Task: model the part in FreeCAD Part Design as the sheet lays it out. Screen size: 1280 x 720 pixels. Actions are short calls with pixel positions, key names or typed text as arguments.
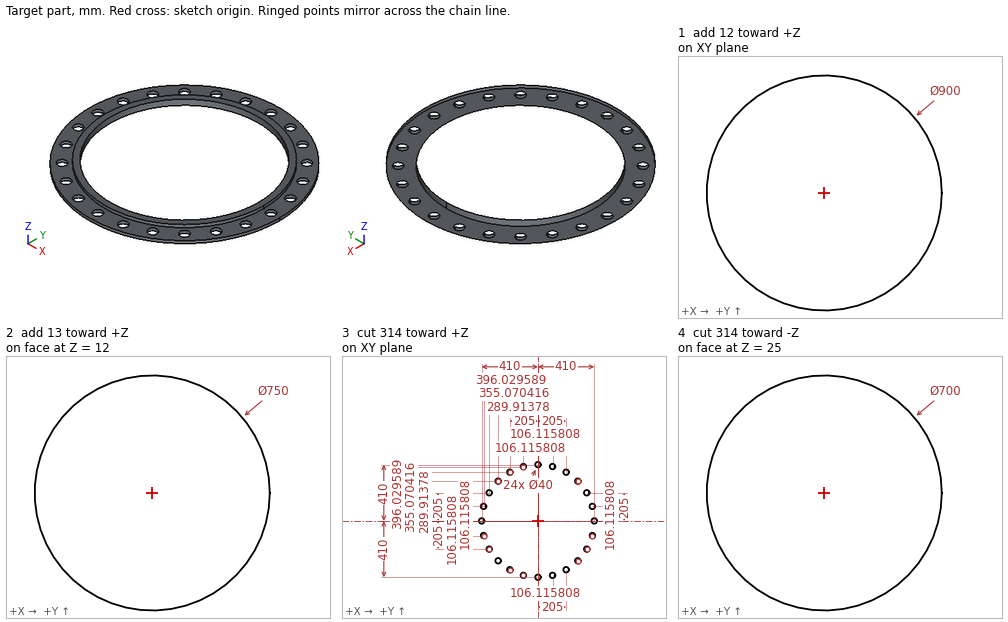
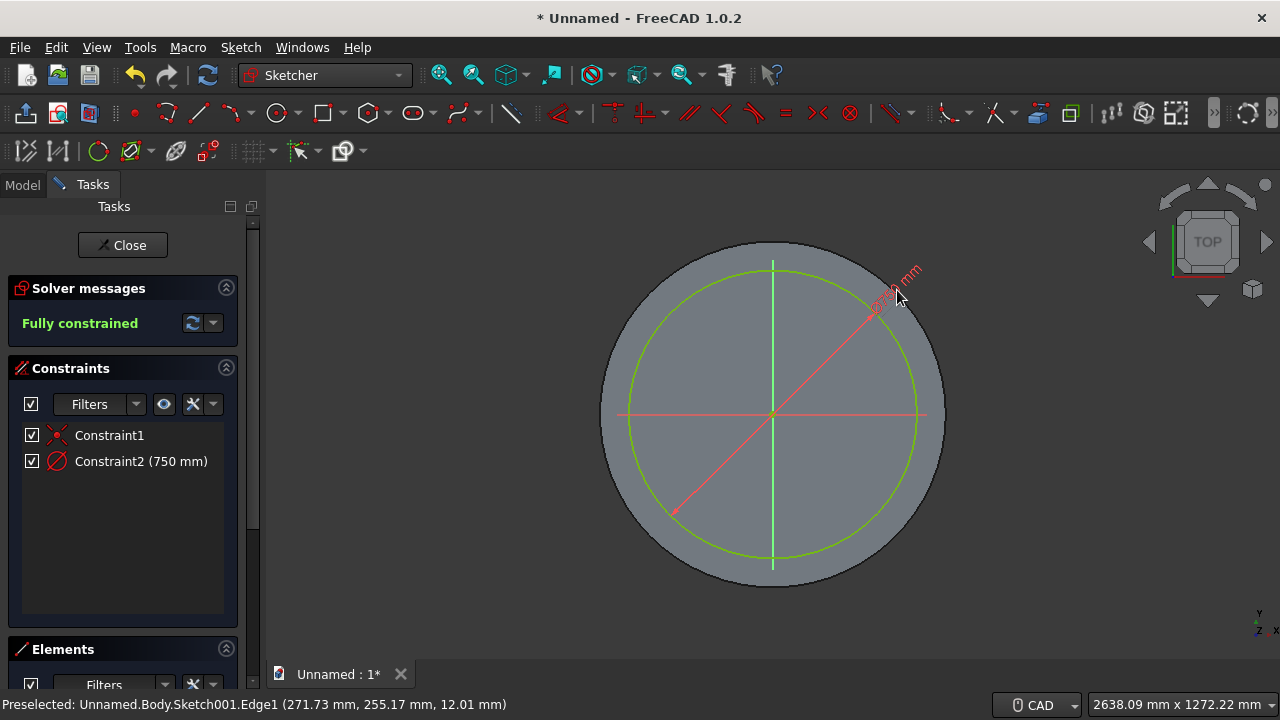
click(123, 245)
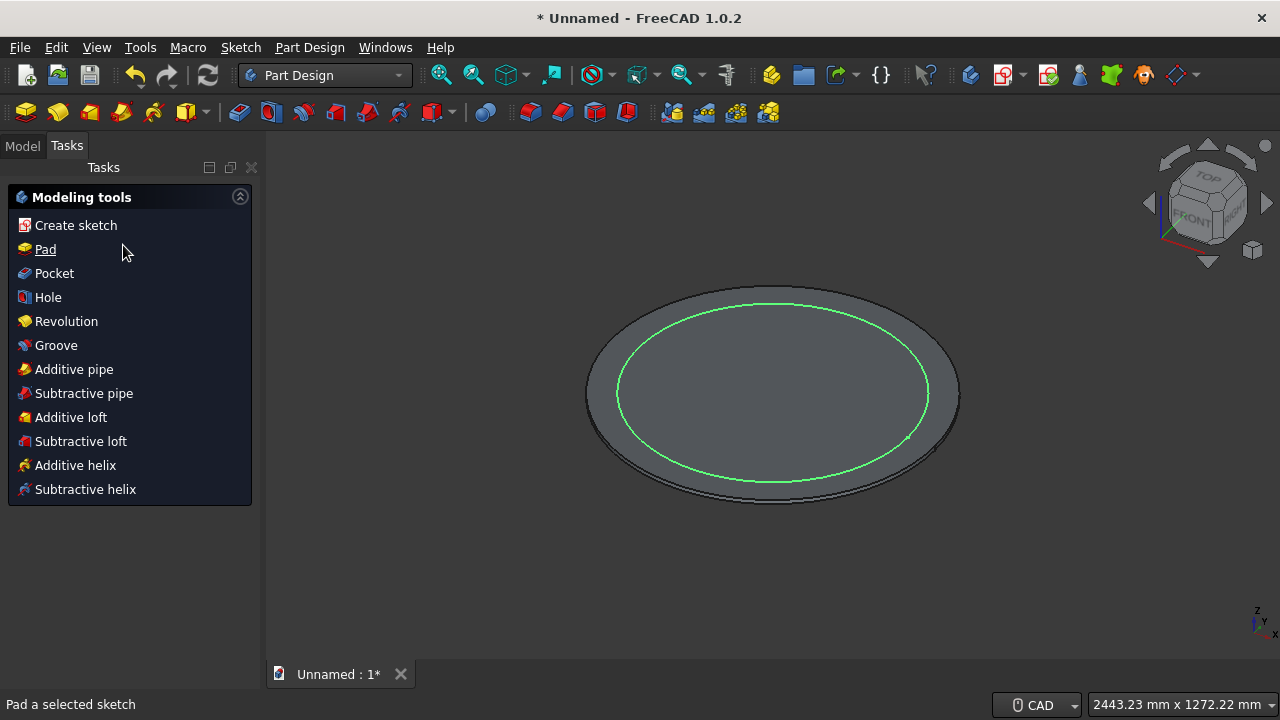
click(26, 112)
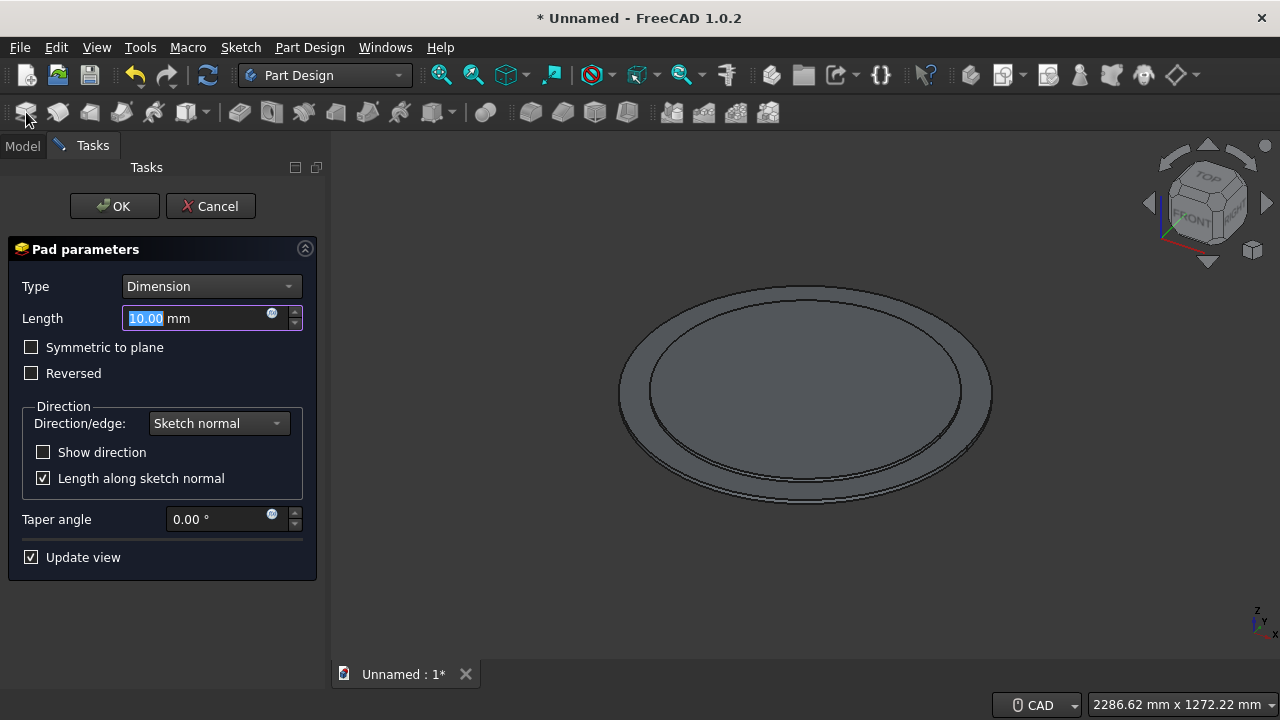
text(13)
key(Tab)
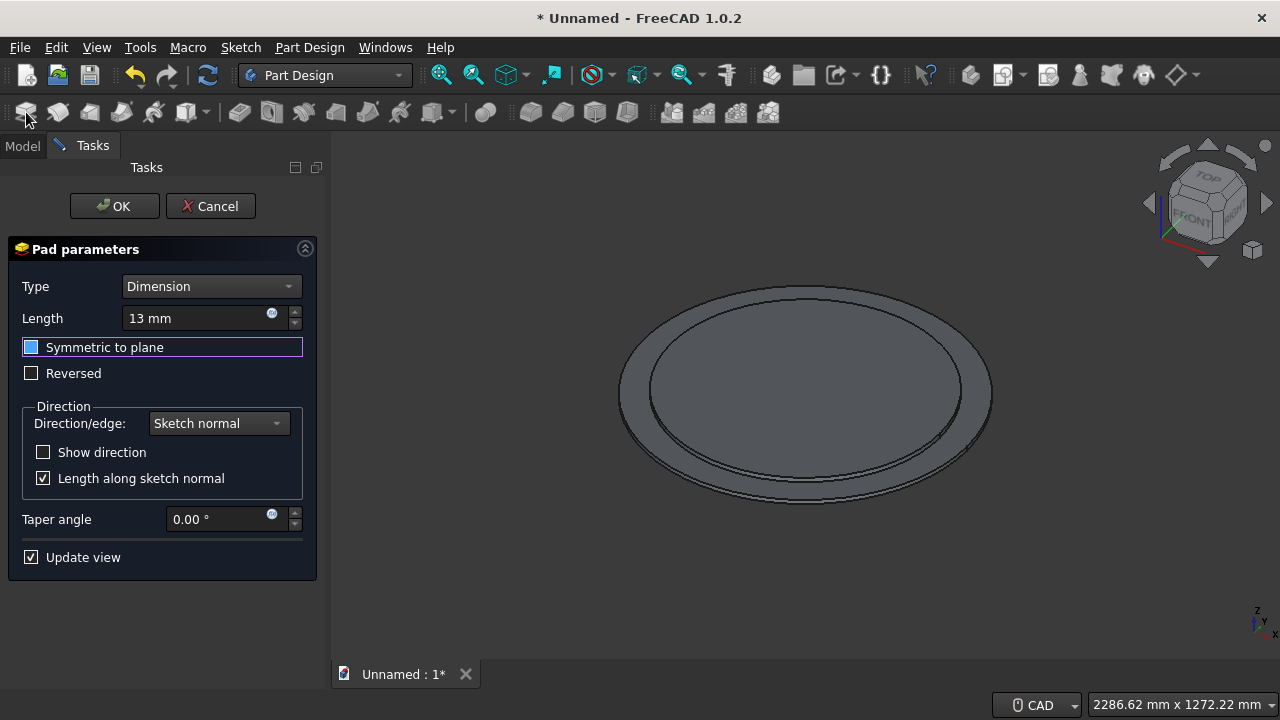
click(115, 206)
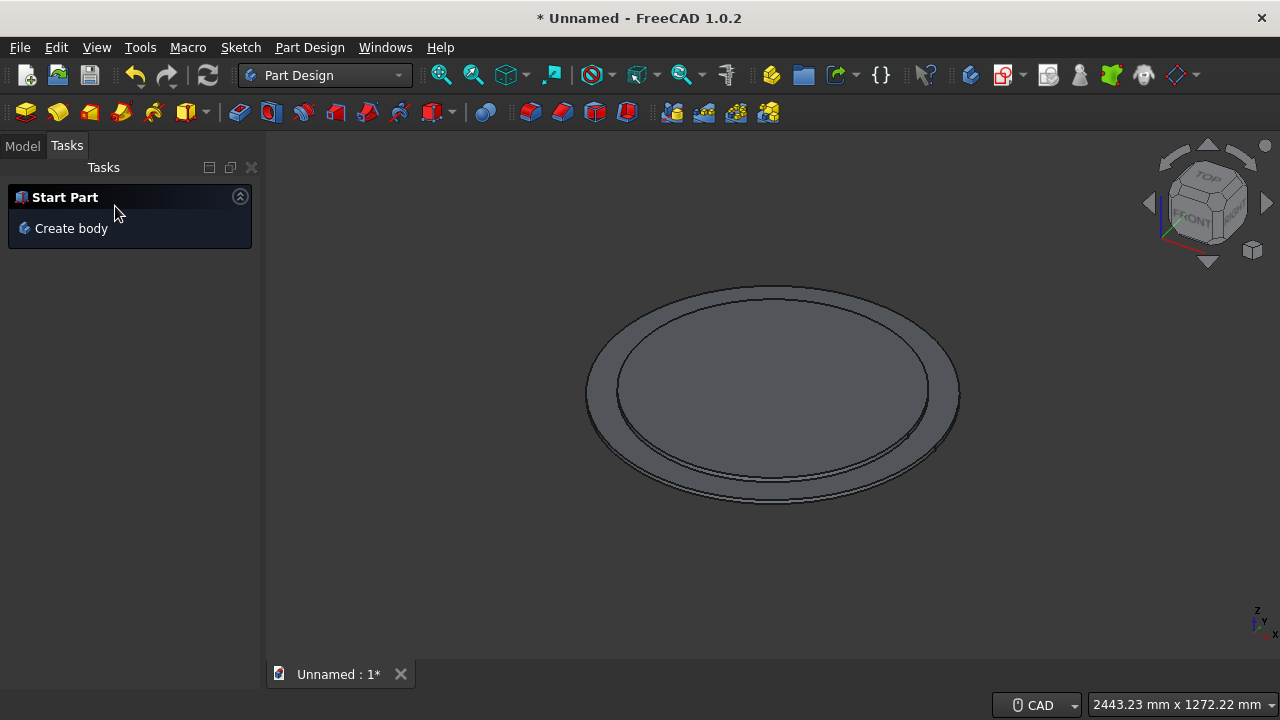
click(1004, 76)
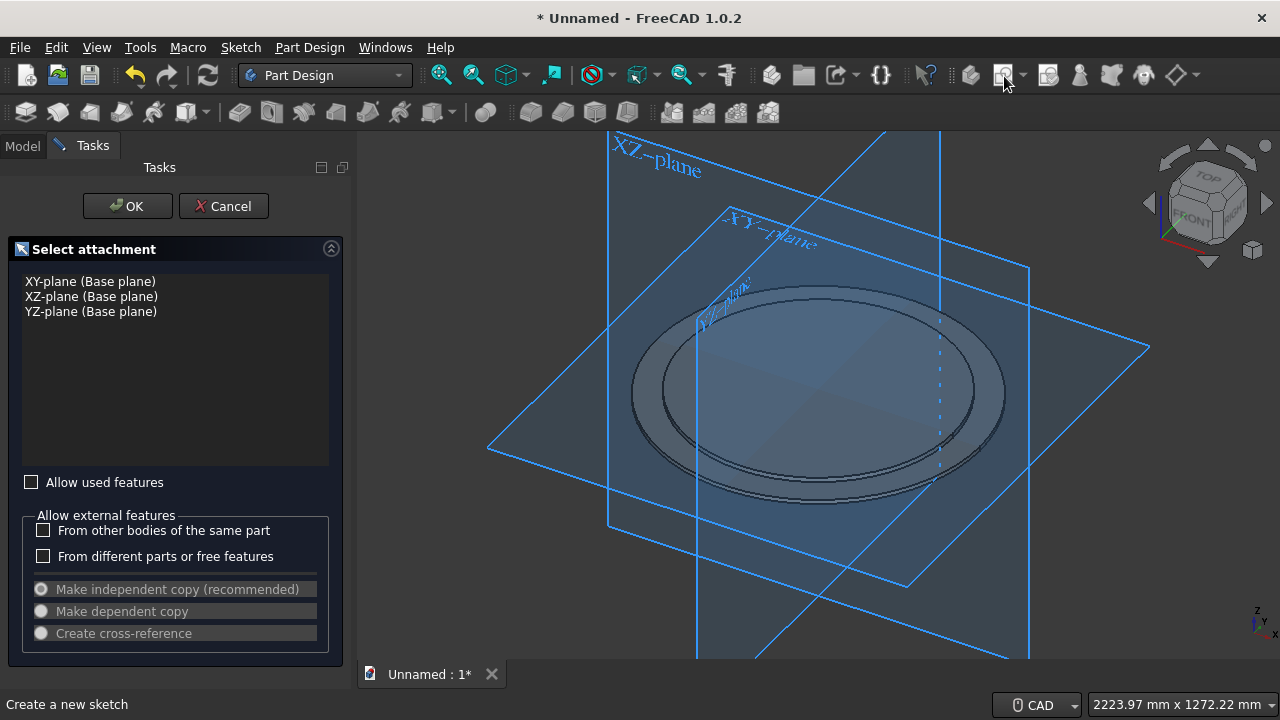
click(82, 282)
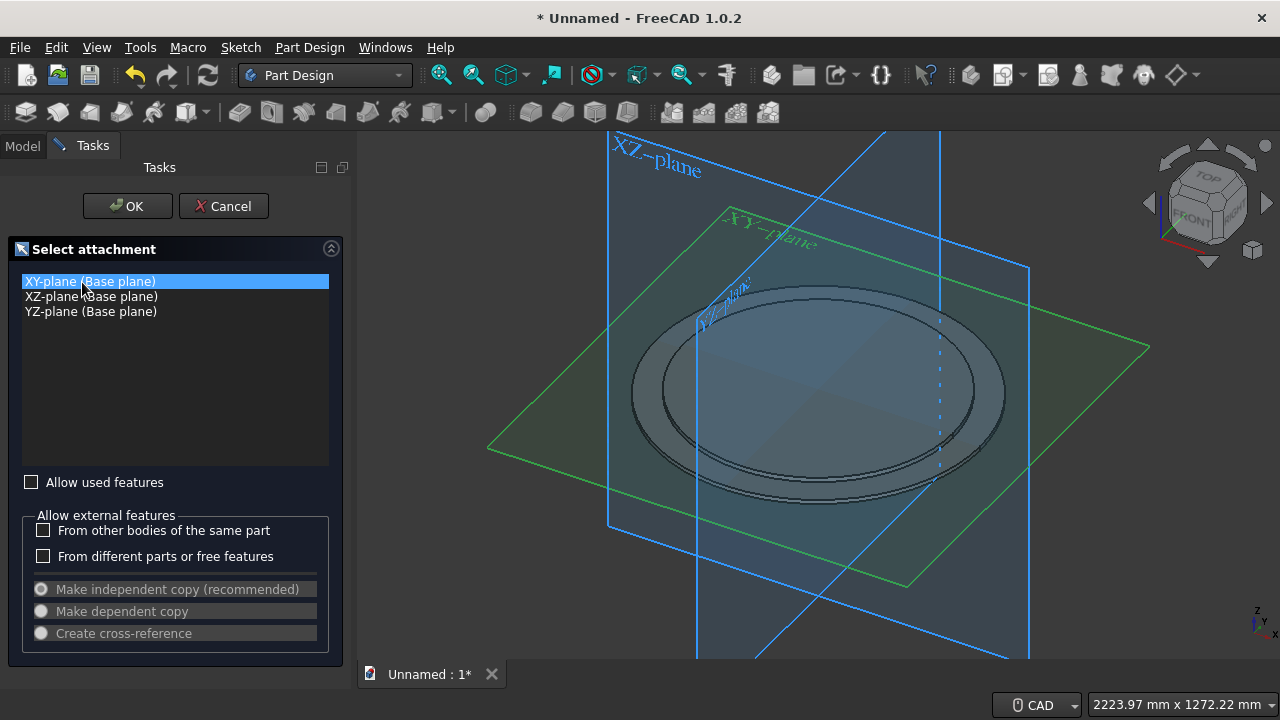
click(128, 206)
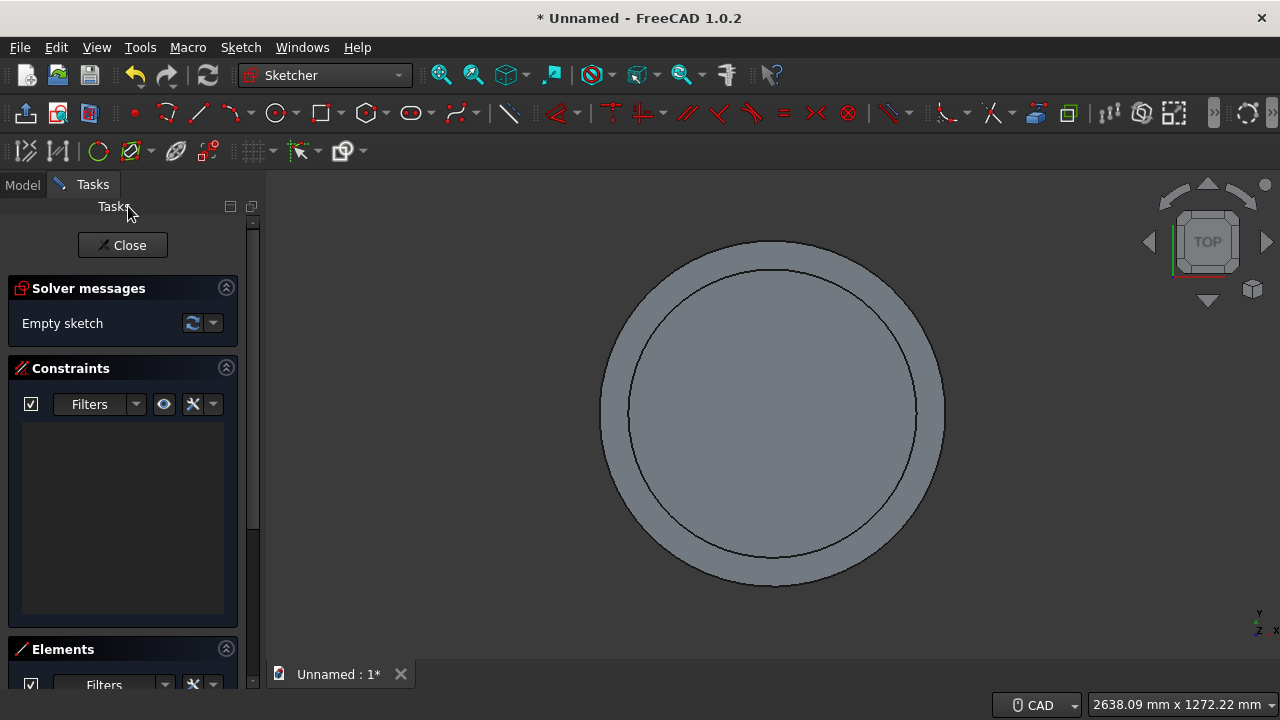
click(90, 114)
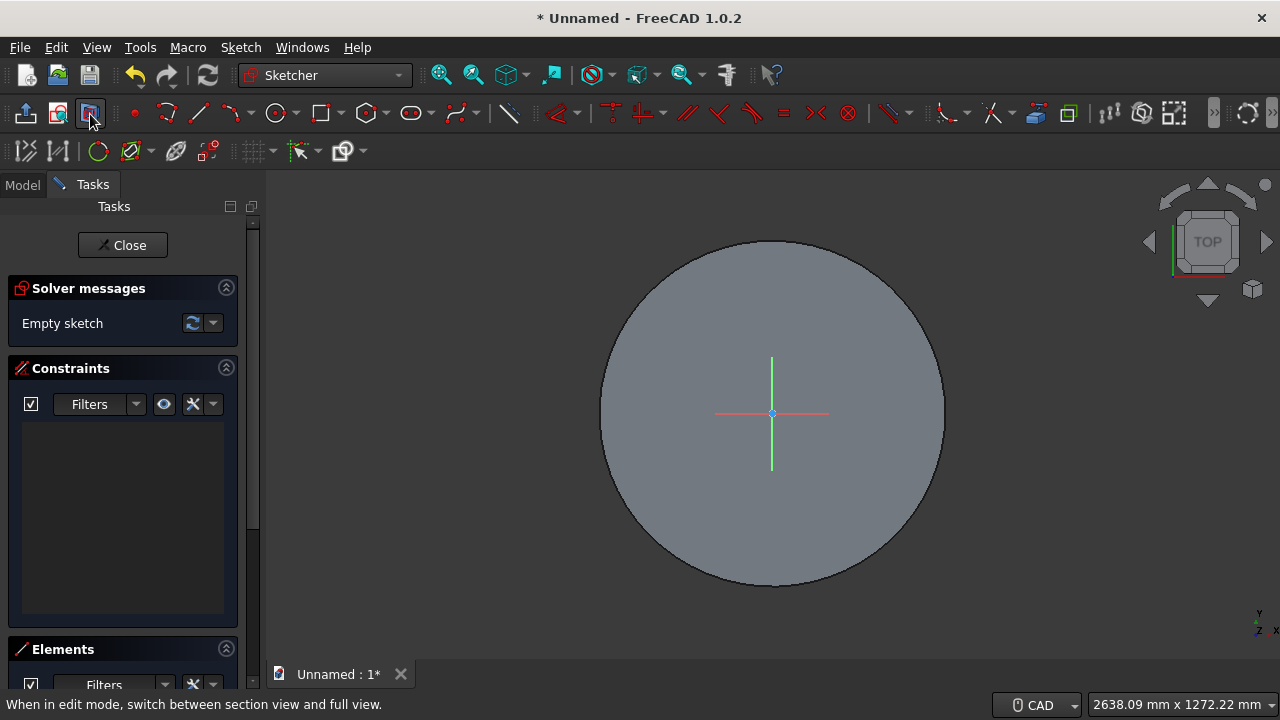
click(276, 114)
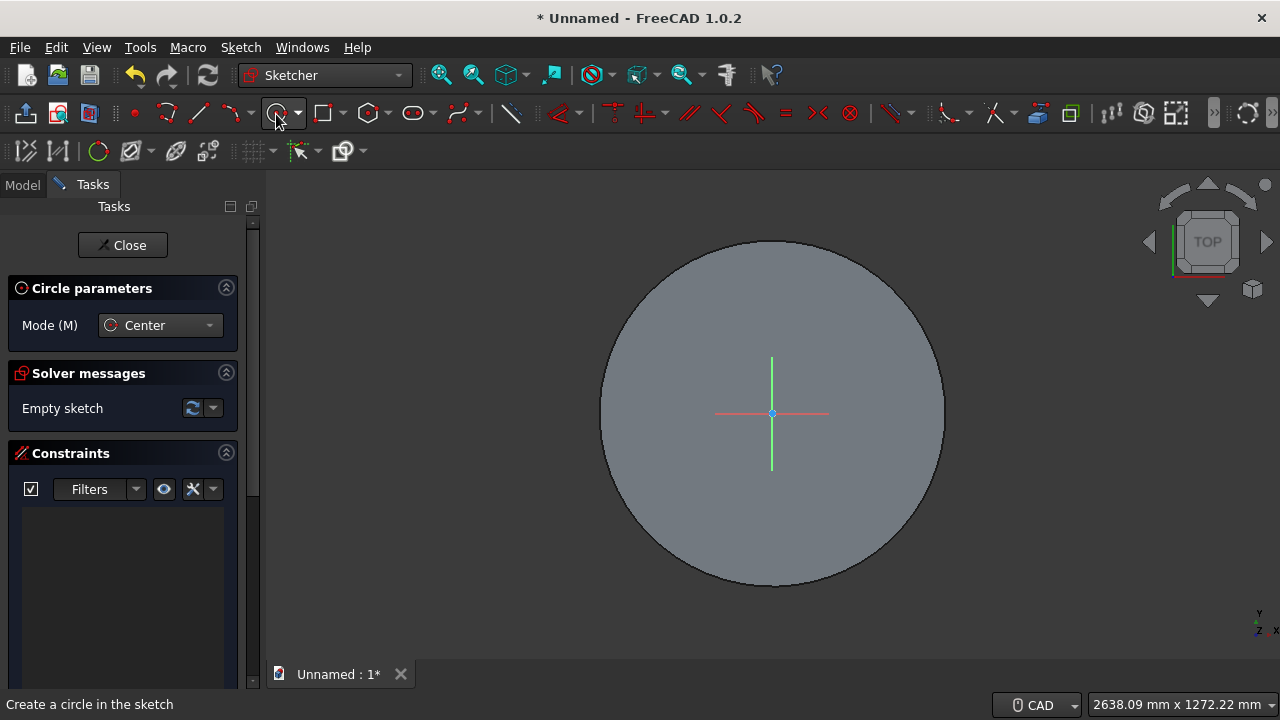
scroll(772, 256, up, 6)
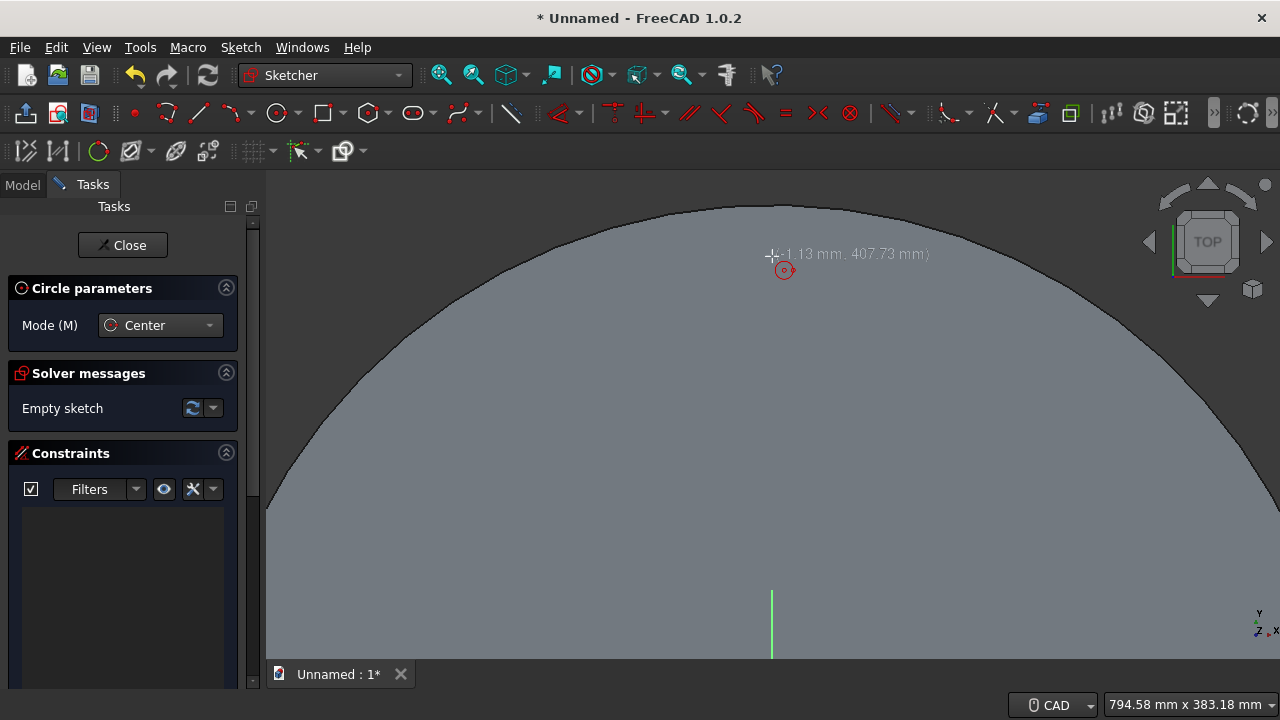
click(772, 256)
click(790, 238)